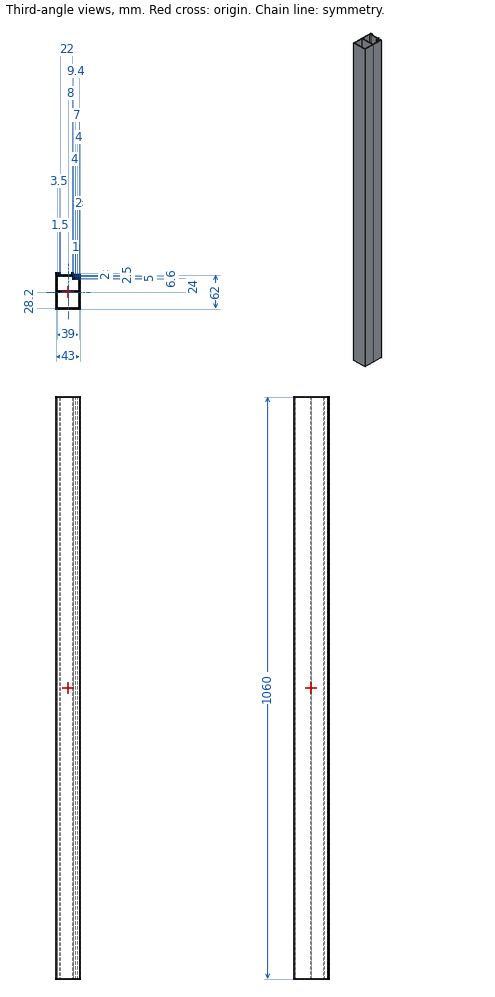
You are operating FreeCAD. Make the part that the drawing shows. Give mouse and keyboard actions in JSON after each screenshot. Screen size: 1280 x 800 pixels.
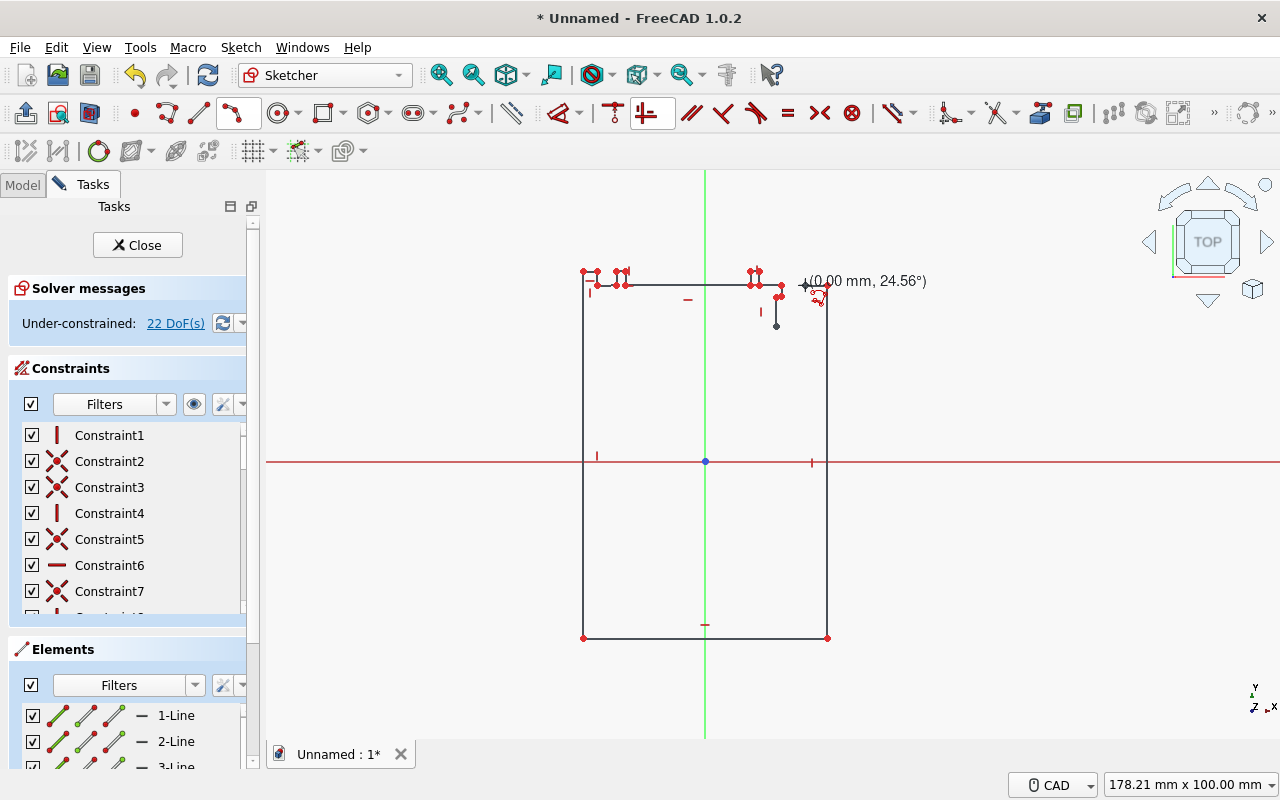
{"action": "scroll", "coordinate": [805, 296], "scroll_direction": "up", "scroll_amount": 2}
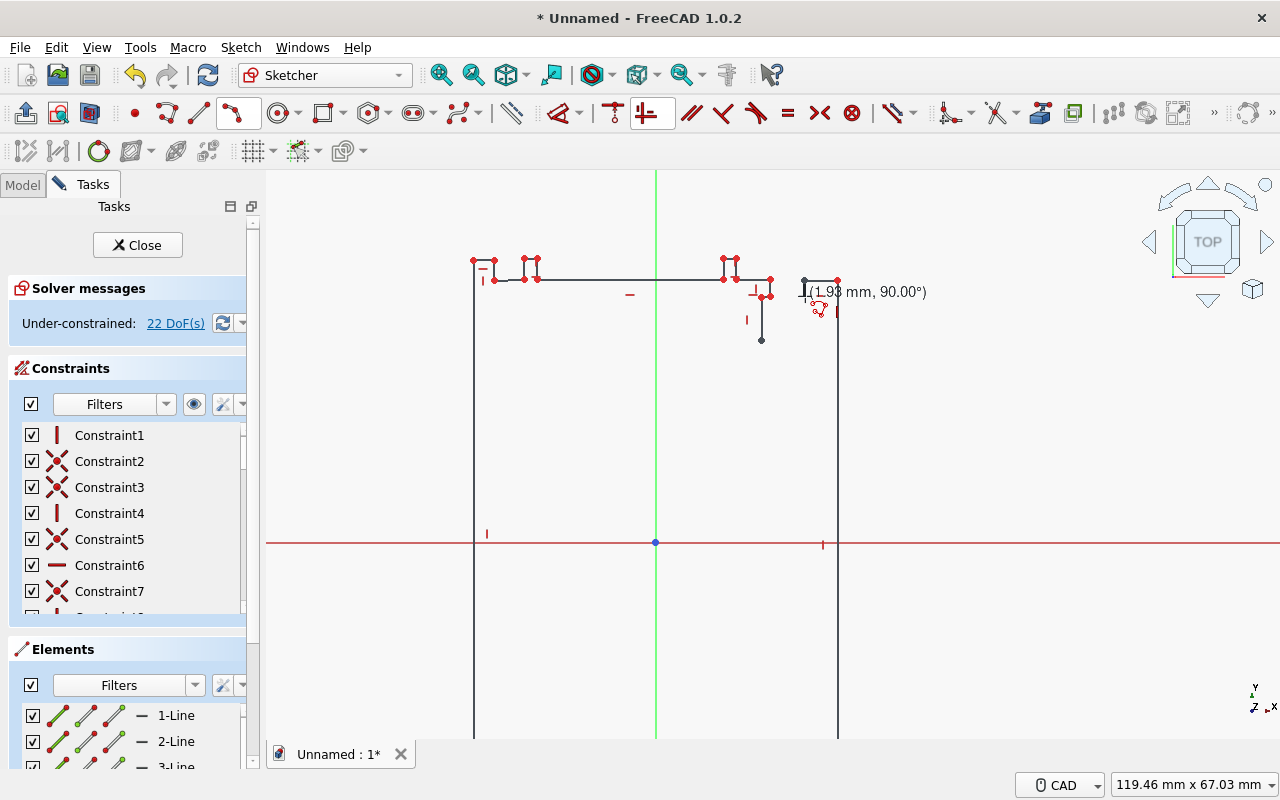
{"action": "left_click", "coordinate": [805, 297]}
{"action": "left_click", "coordinate": [821, 297]}
{"action": "left_click", "coordinate": [821, 339]}
{"action": "left_click", "coordinate": [762, 341]}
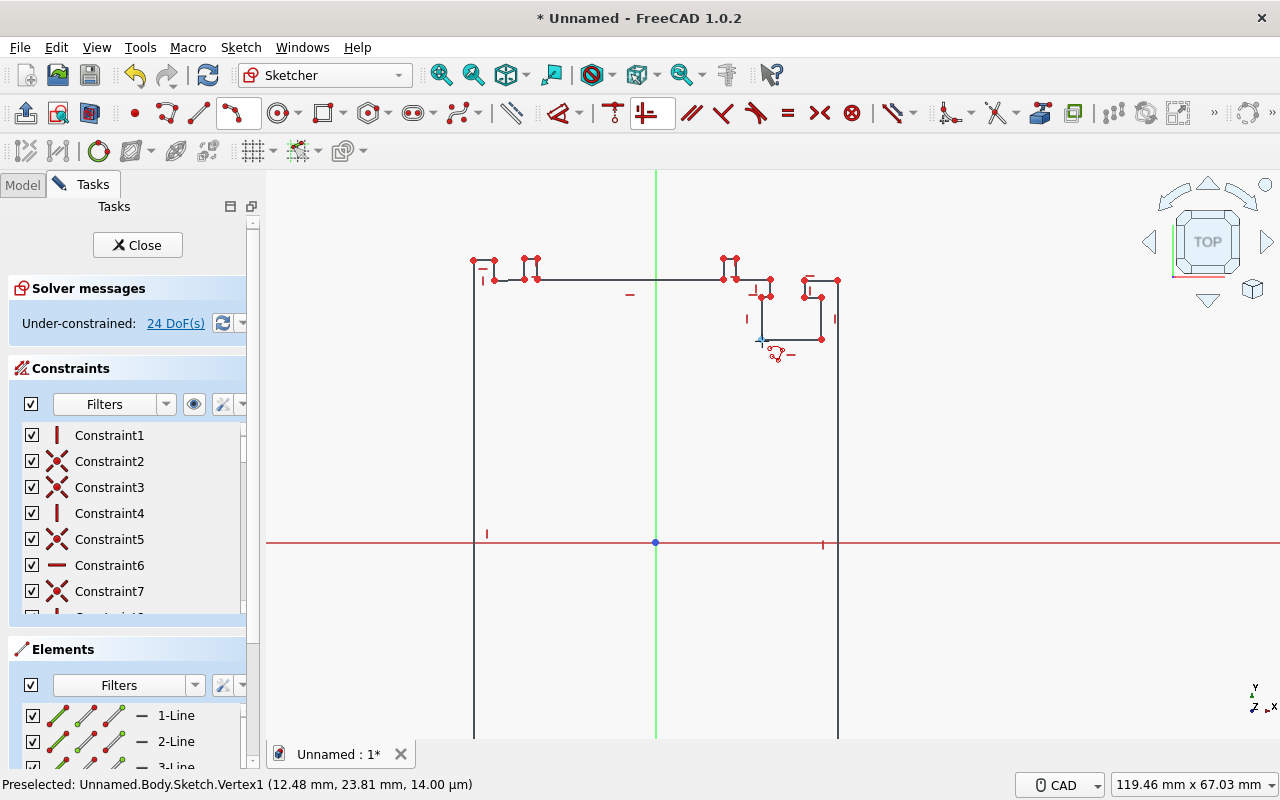
{"action": "left_click", "coordinate": [324, 114]}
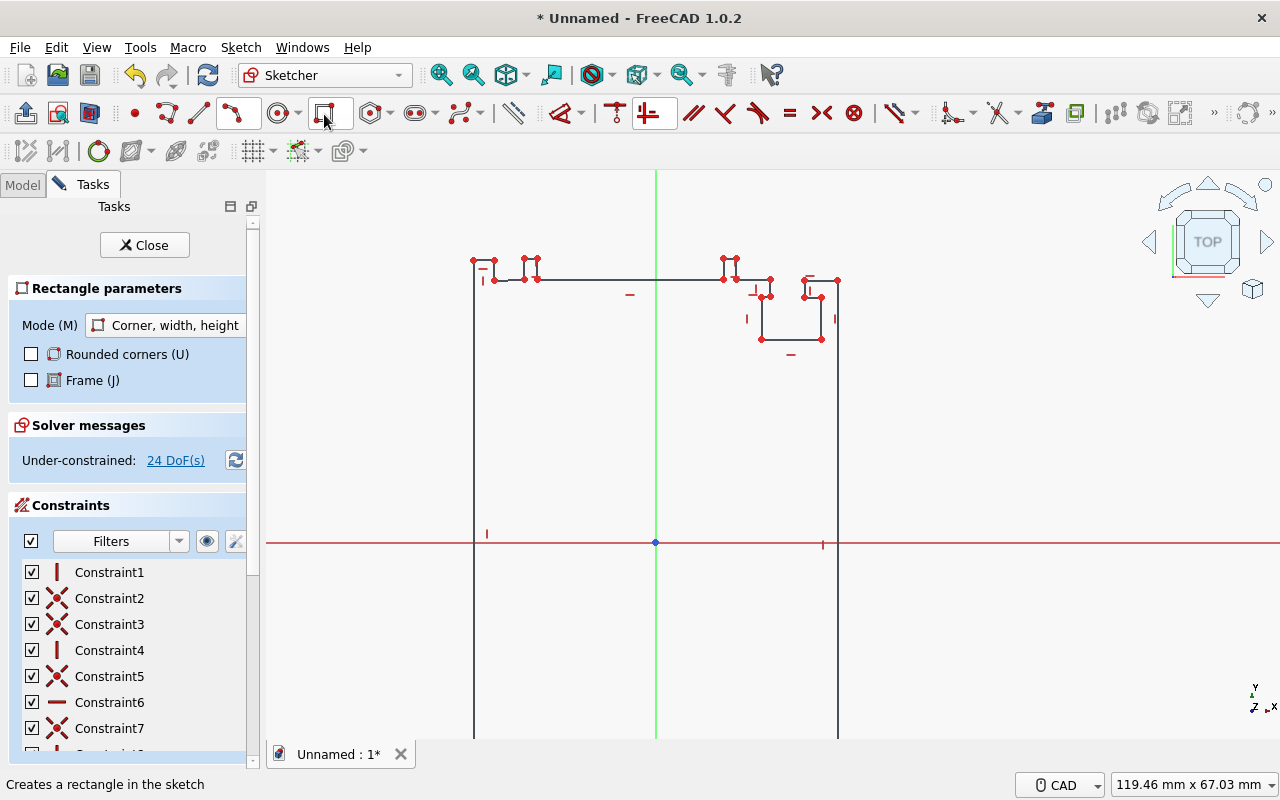
{"action": "scroll", "coordinate": [490, 550], "scroll_direction": "up", "scroll_amount": 5}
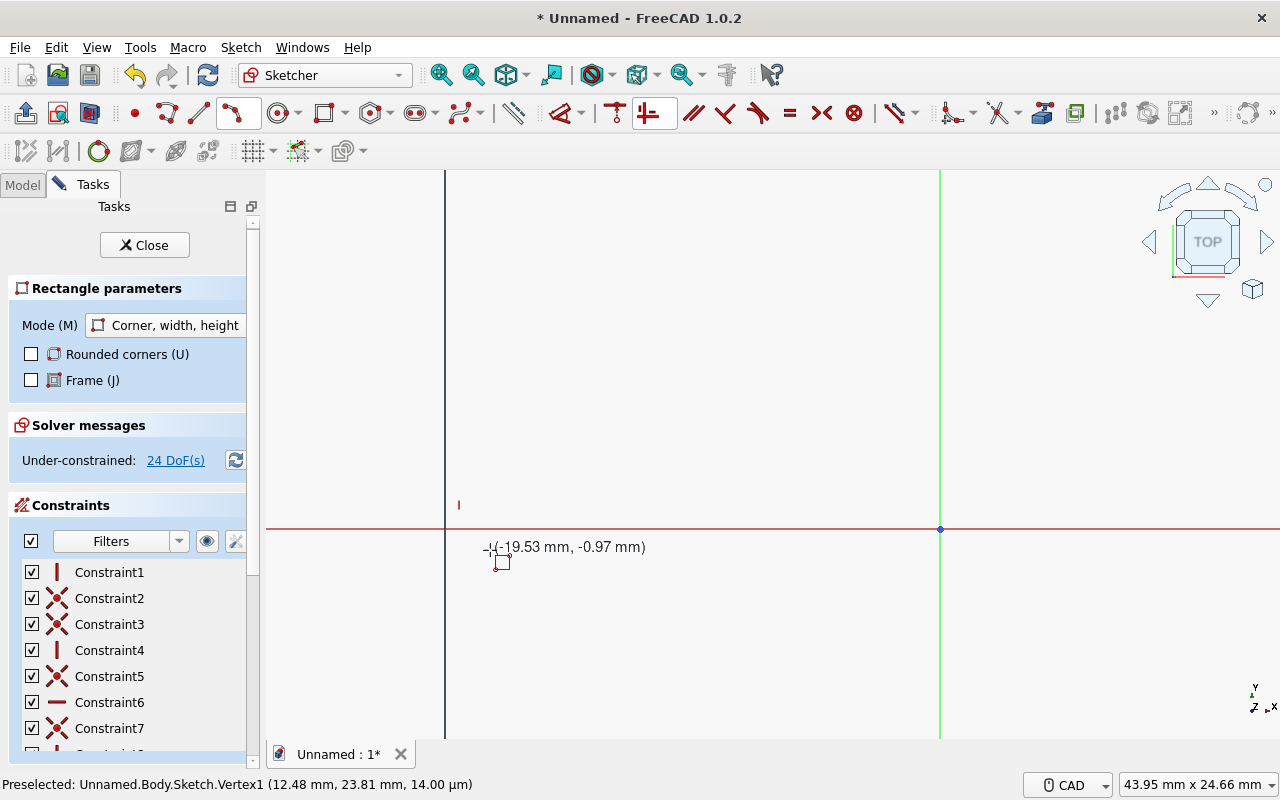
{"action": "left_click", "coordinate": [490, 548]}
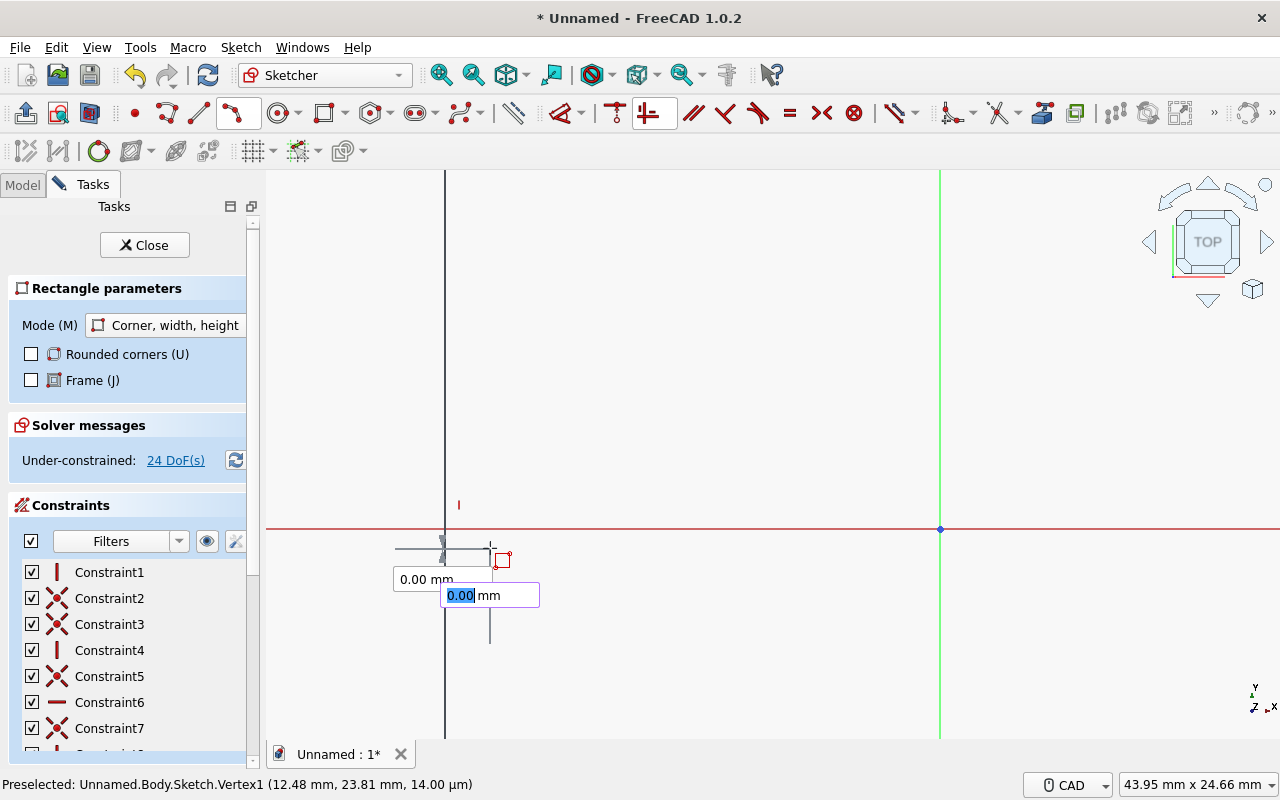
{"action": "scroll", "coordinate": [627, 439], "scroll_direction": "down", "scroll_amount": 7}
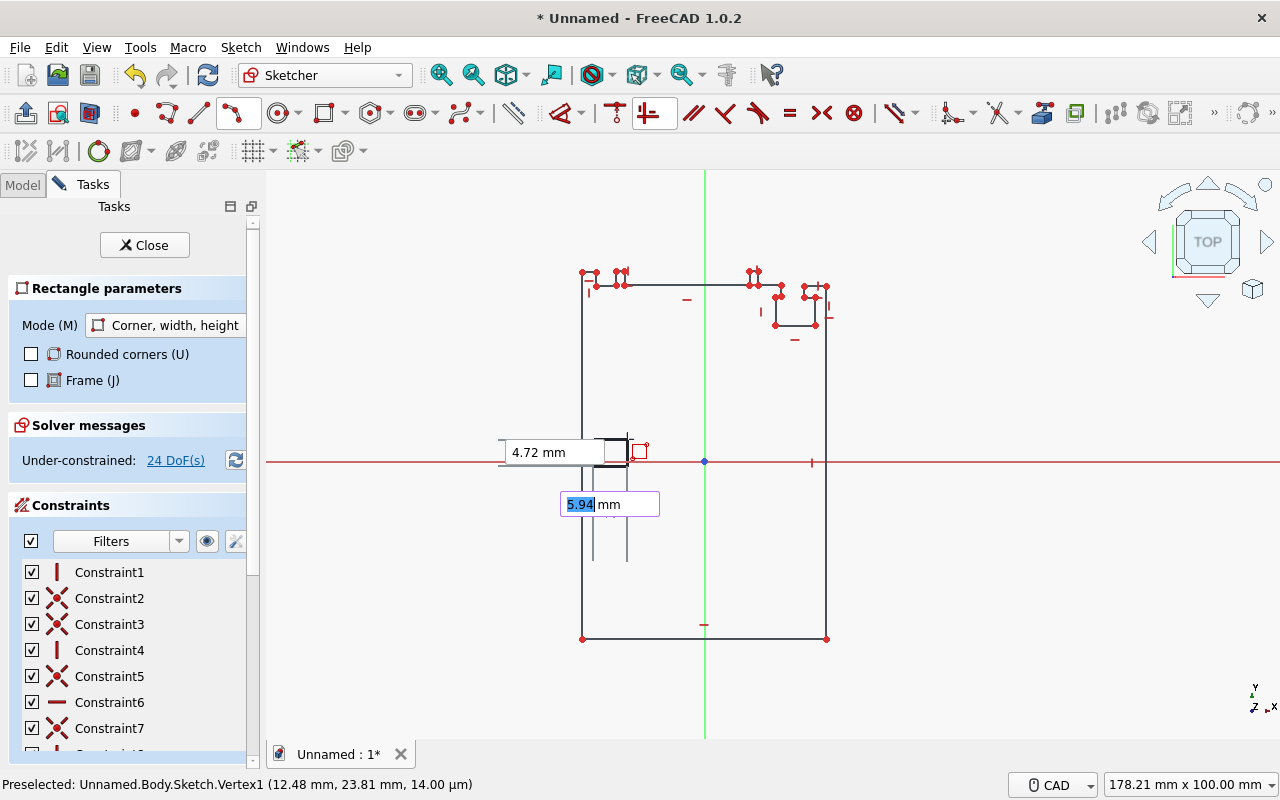
{"action": "scroll", "coordinate": [815, 627], "scroll_direction": "up", "scroll_amount": 2}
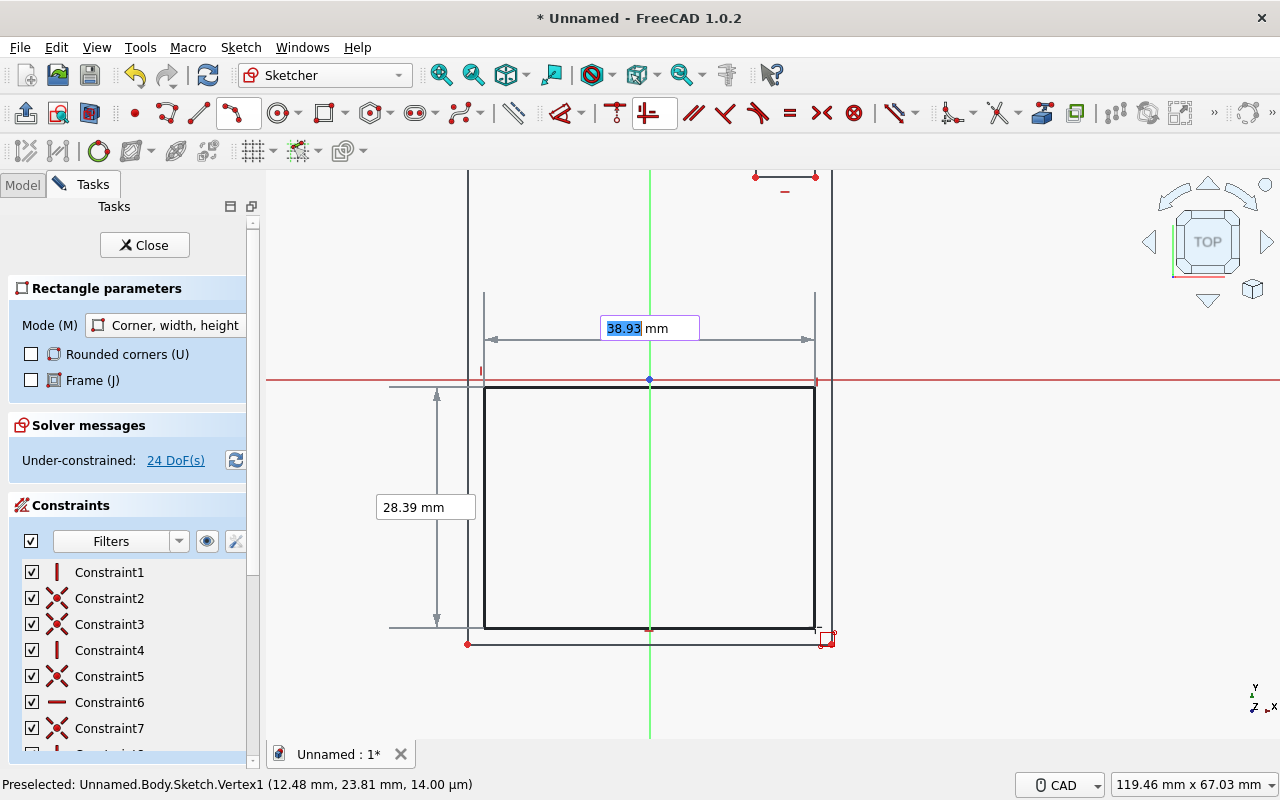
{"action": "left_click", "coordinate": [815, 626]}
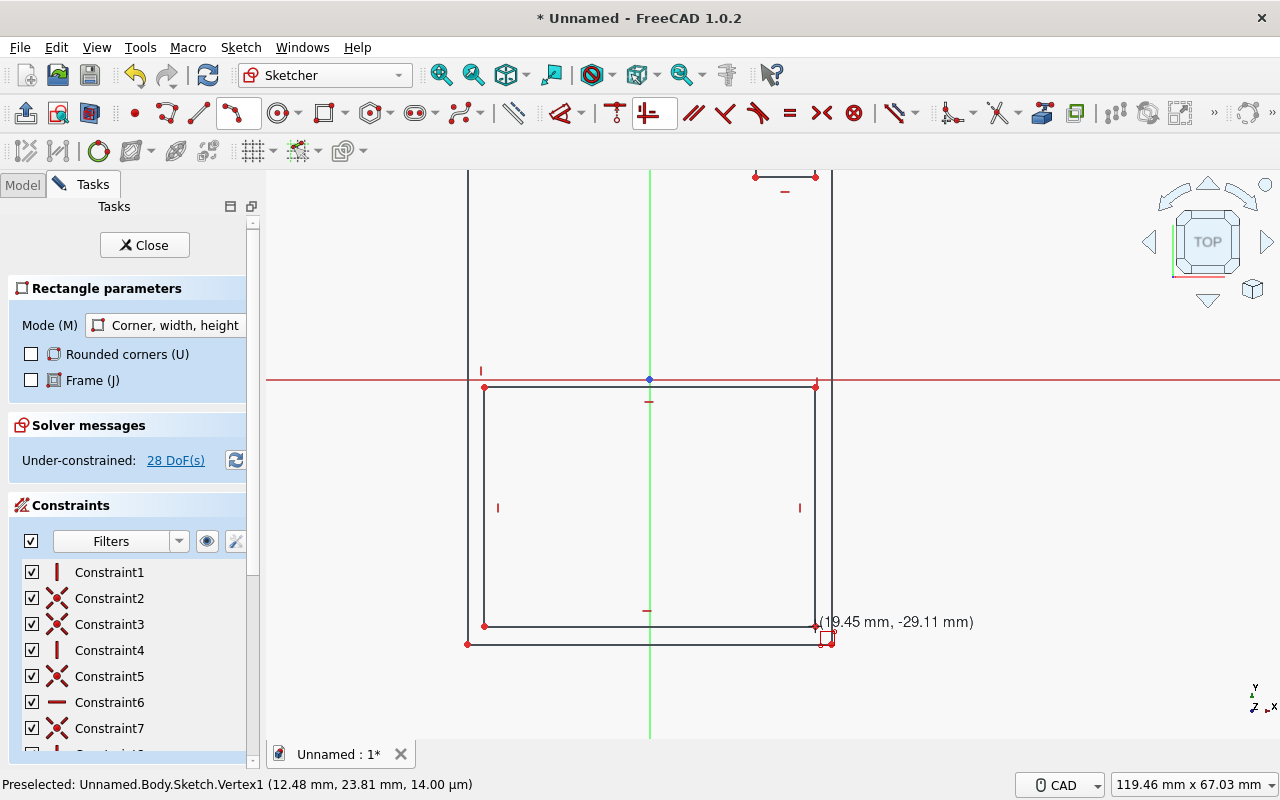
{"action": "left_click", "coordinate": [168, 114]}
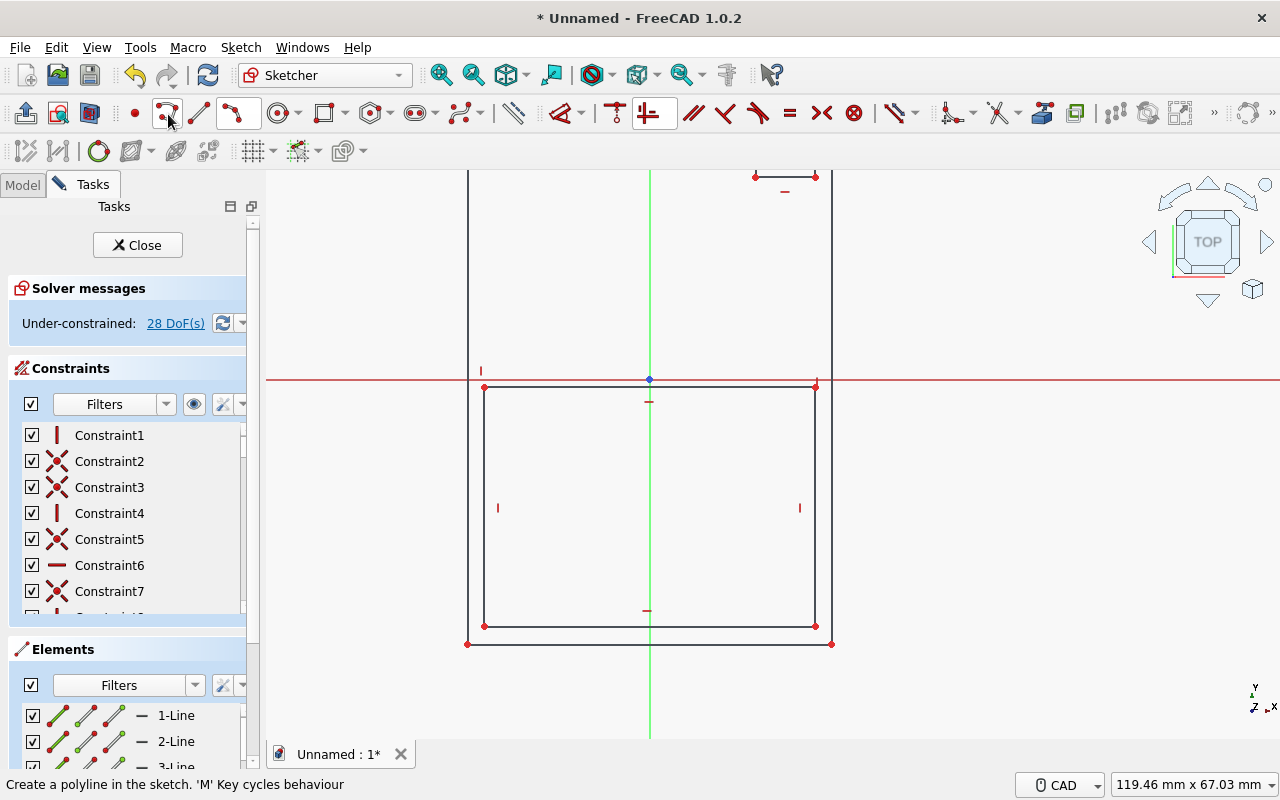
{"action": "scroll", "coordinate": [815, 373], "scroll_direction": "up", "scroll_amount": 5}